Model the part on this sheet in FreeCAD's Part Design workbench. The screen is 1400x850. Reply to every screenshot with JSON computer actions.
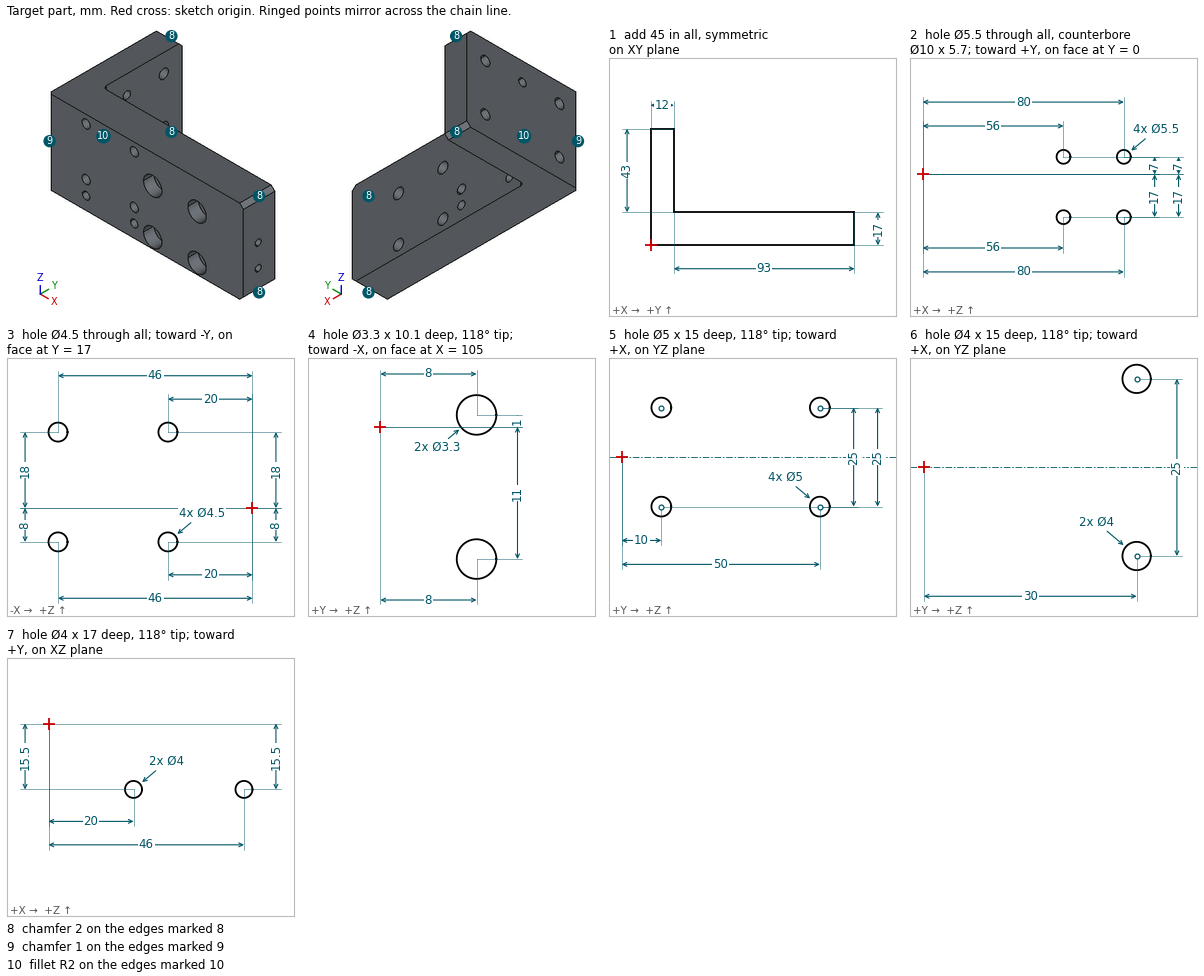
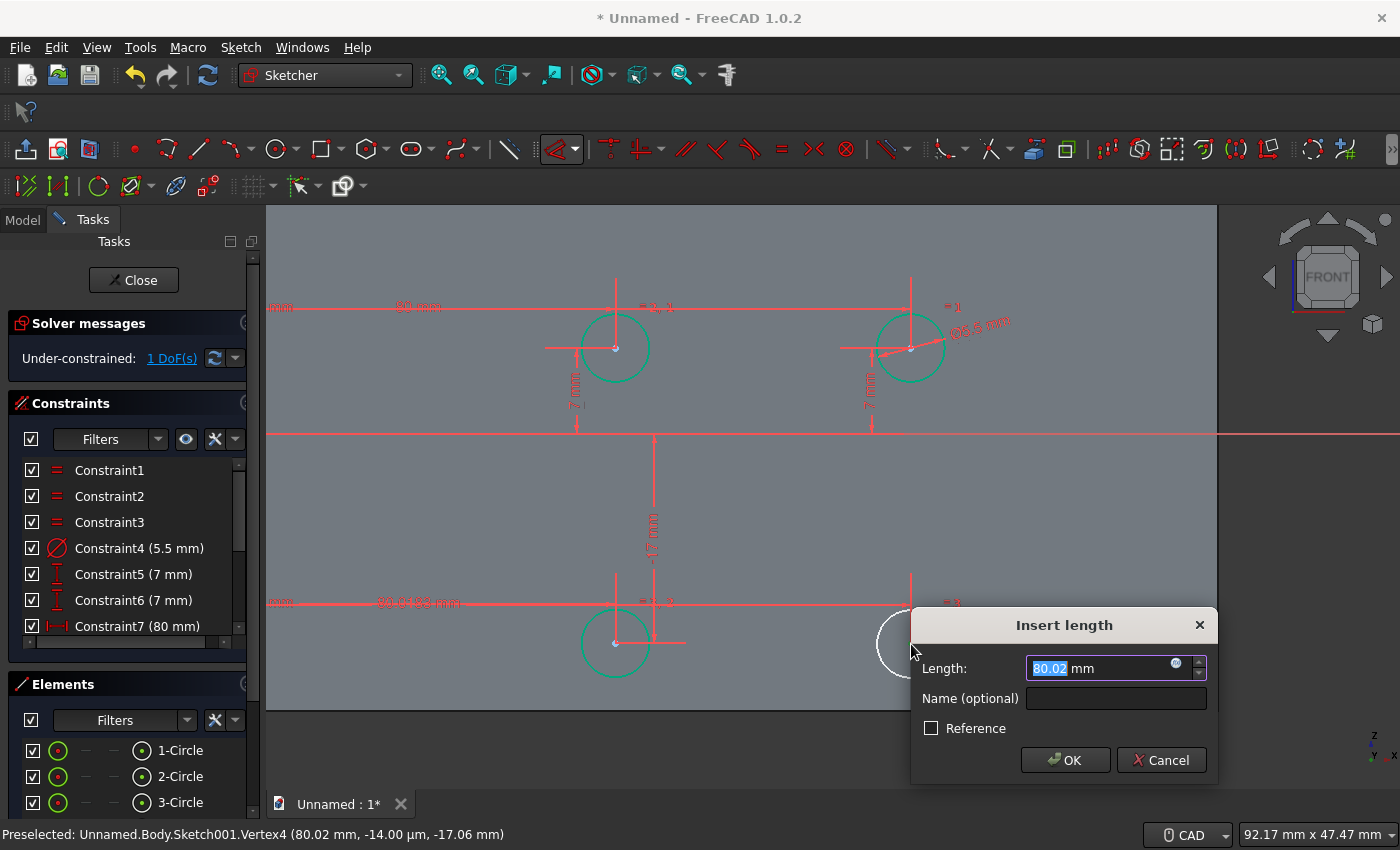
{"action": "type", "text": "80"}
{"action": "key", "text": "Return"}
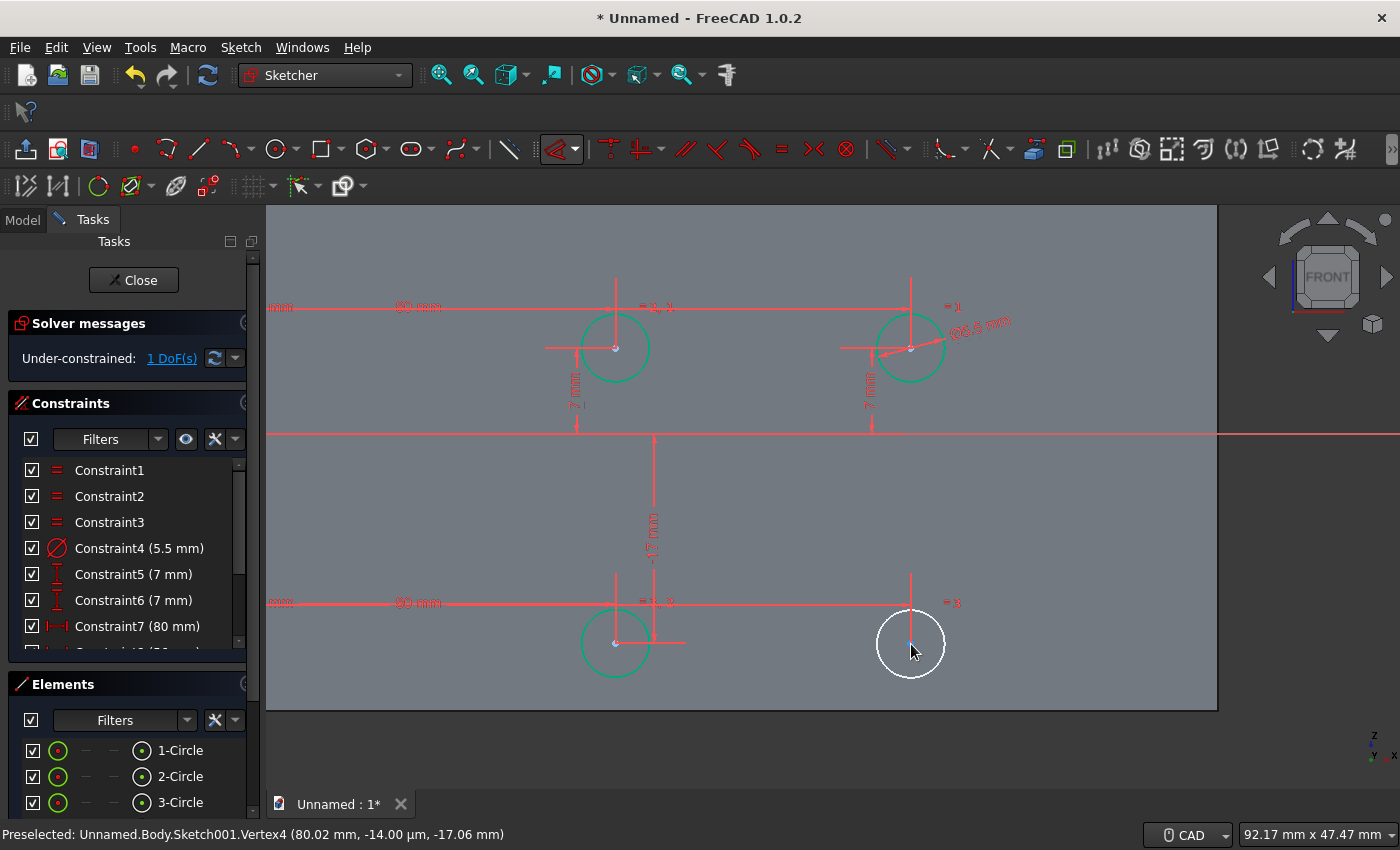
{"action": "left_click", "coordinate": [911, 644]}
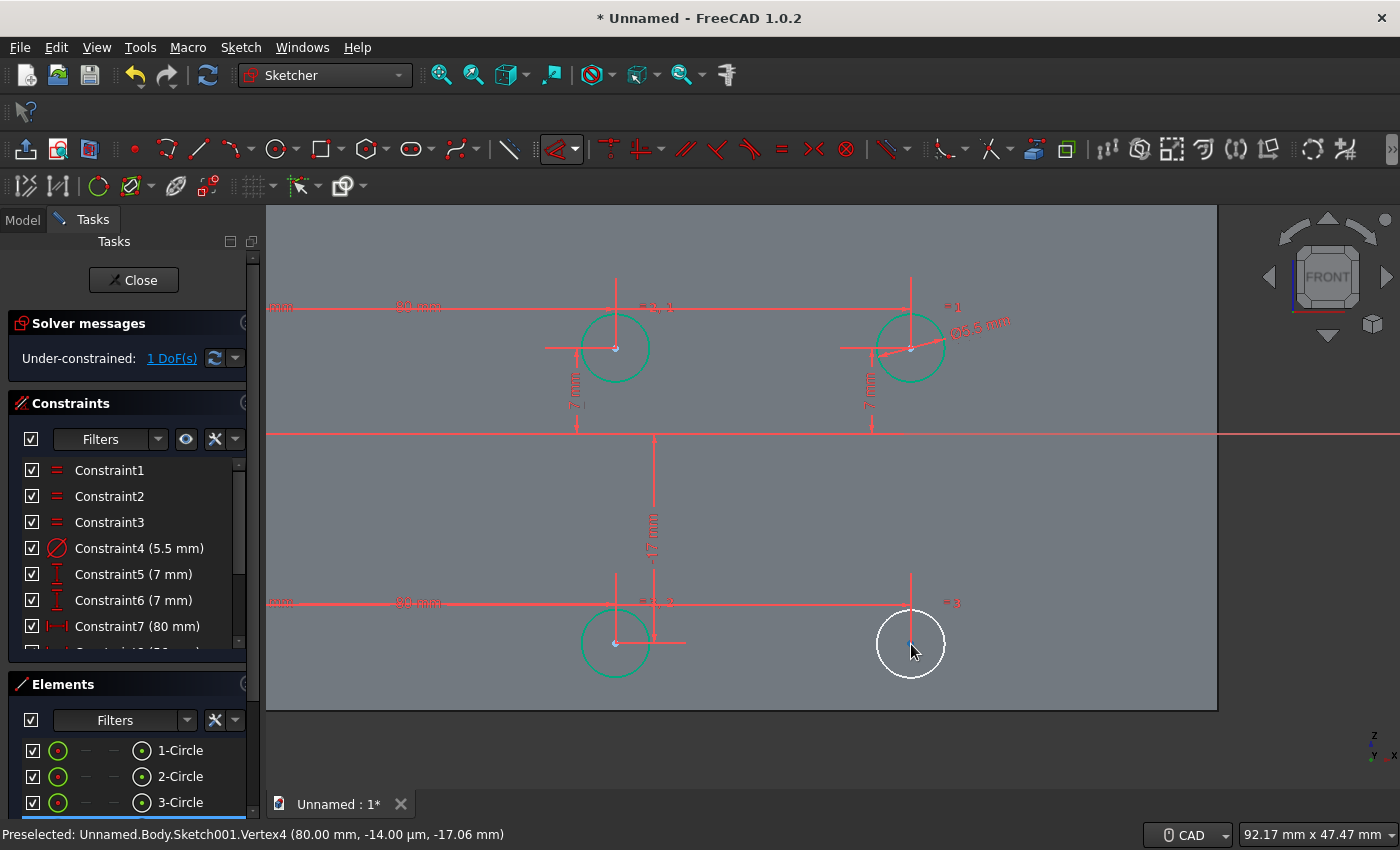
{"action": "key", "text": "i"}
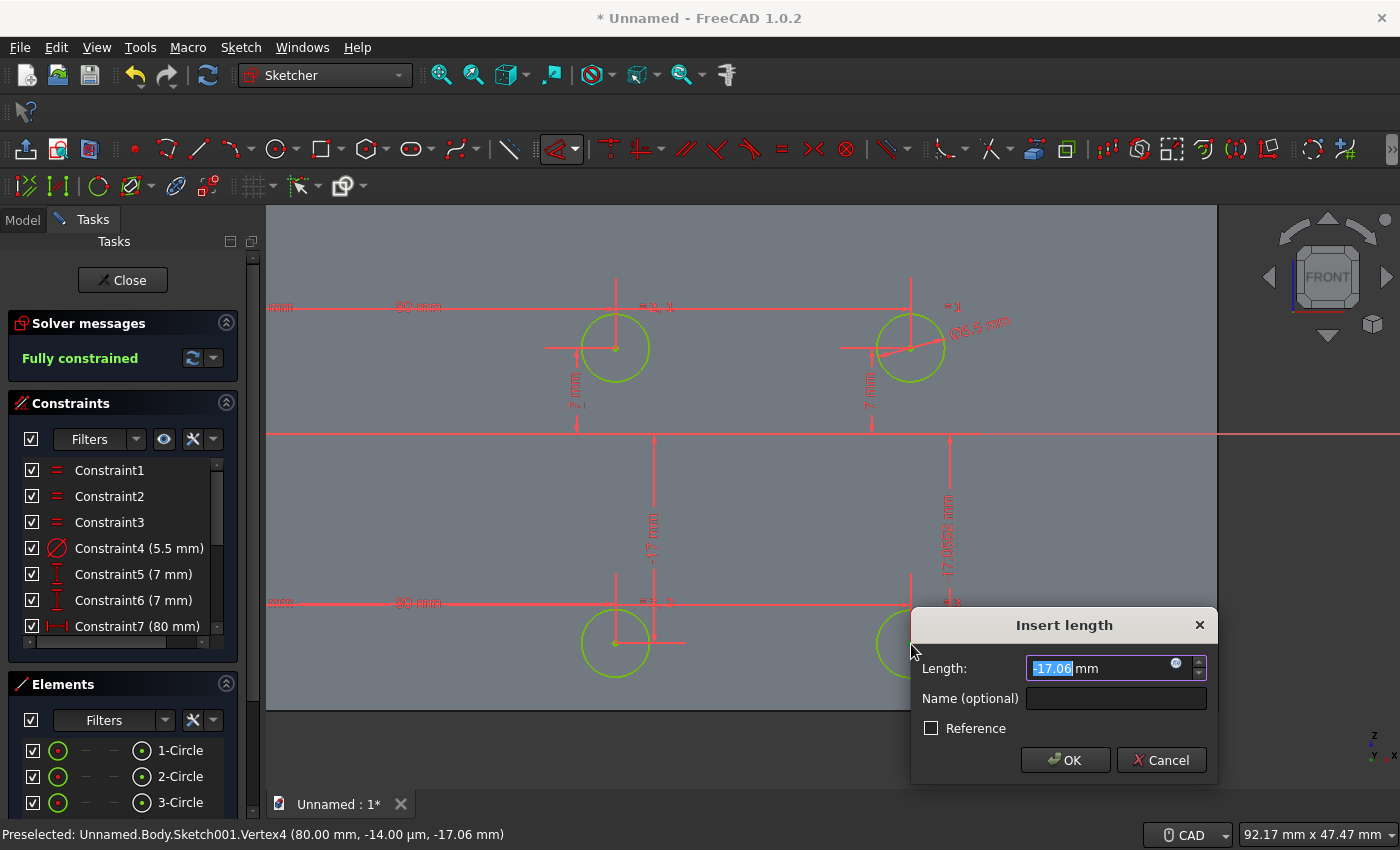
{"action": "type", "text": "-17"}
{"action": "key", "text": "Return"}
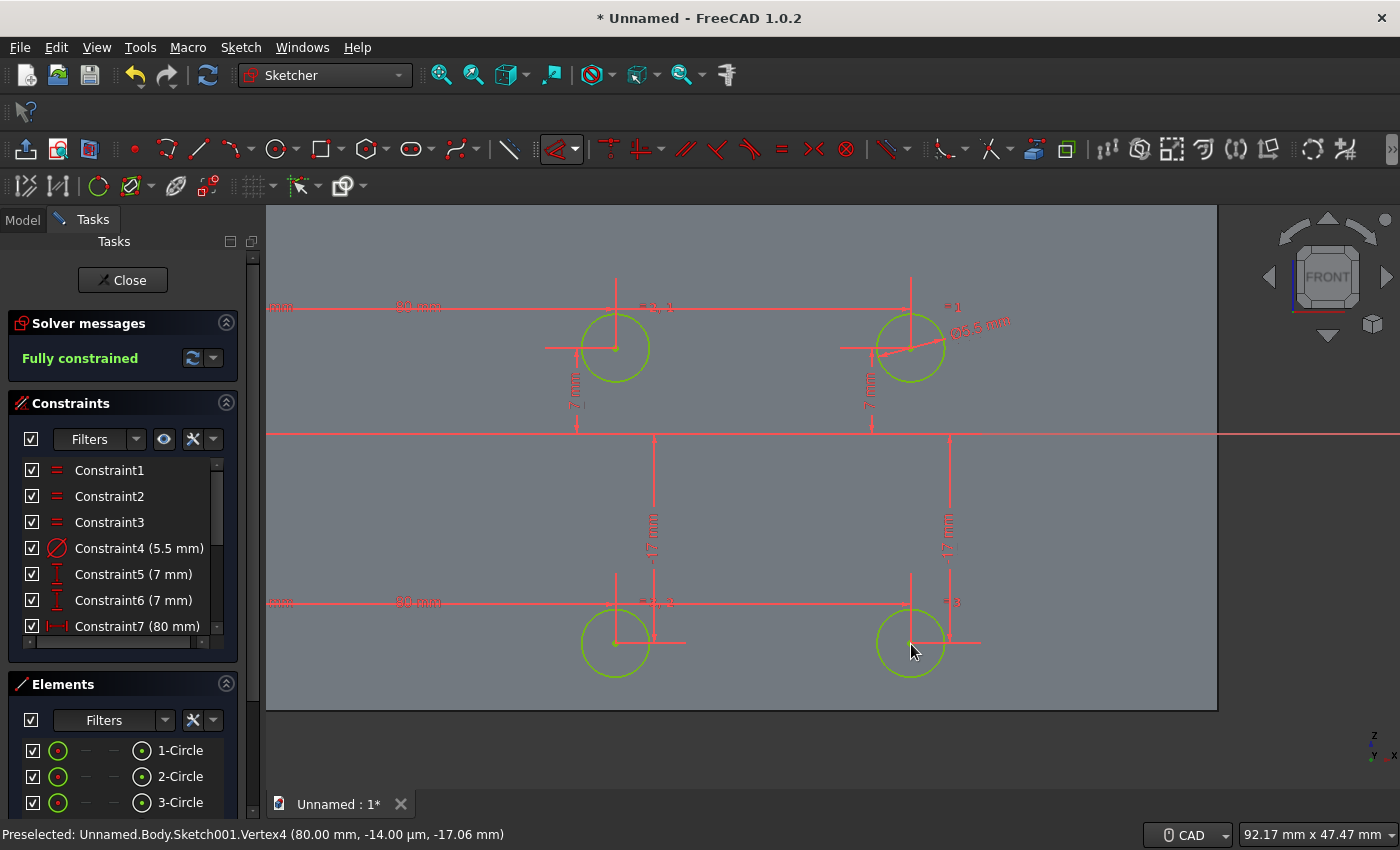
{"action": "left_click", "coordinate": [123, 280]}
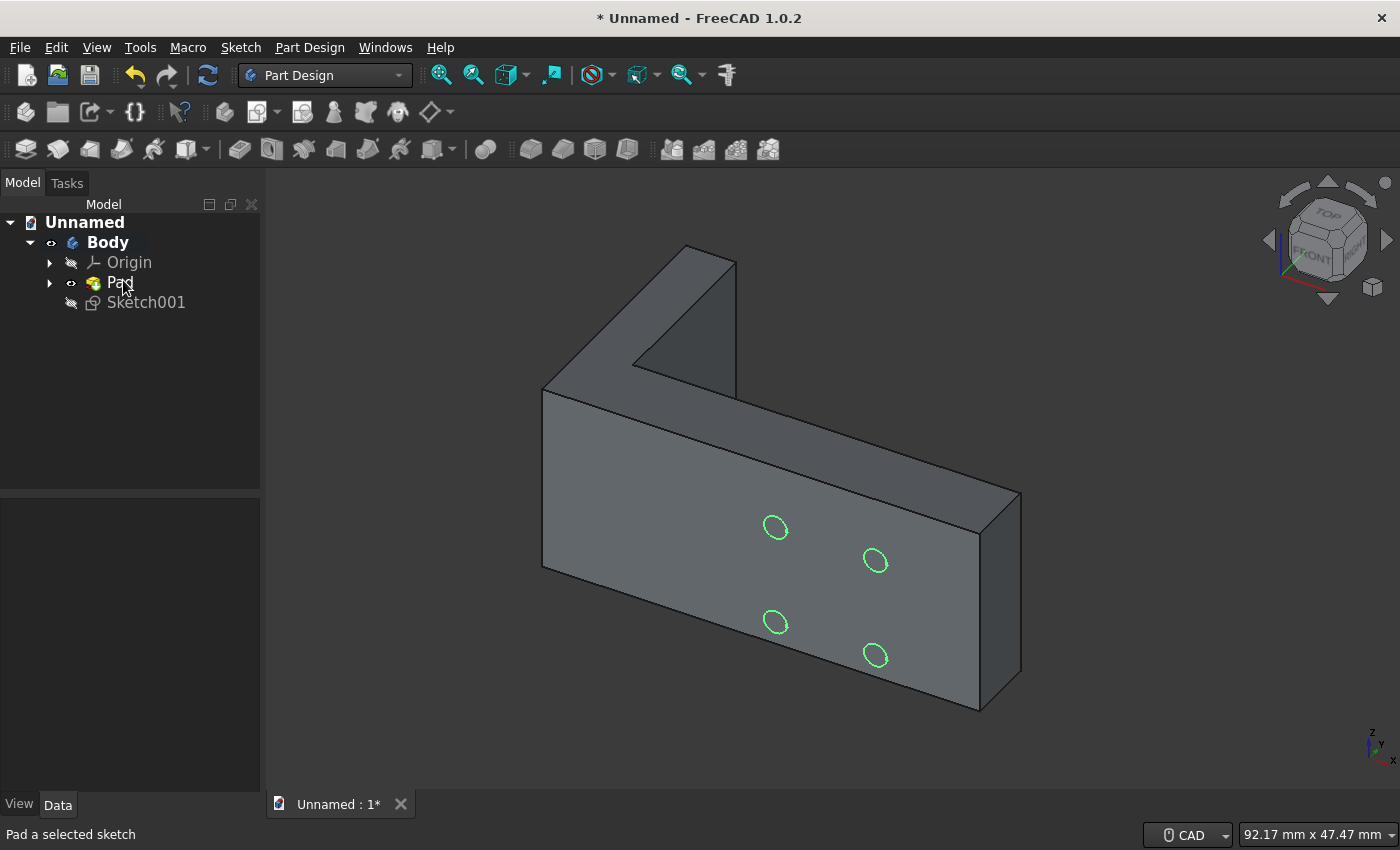
{"action": "left_click", "coordinate": [272, 150]}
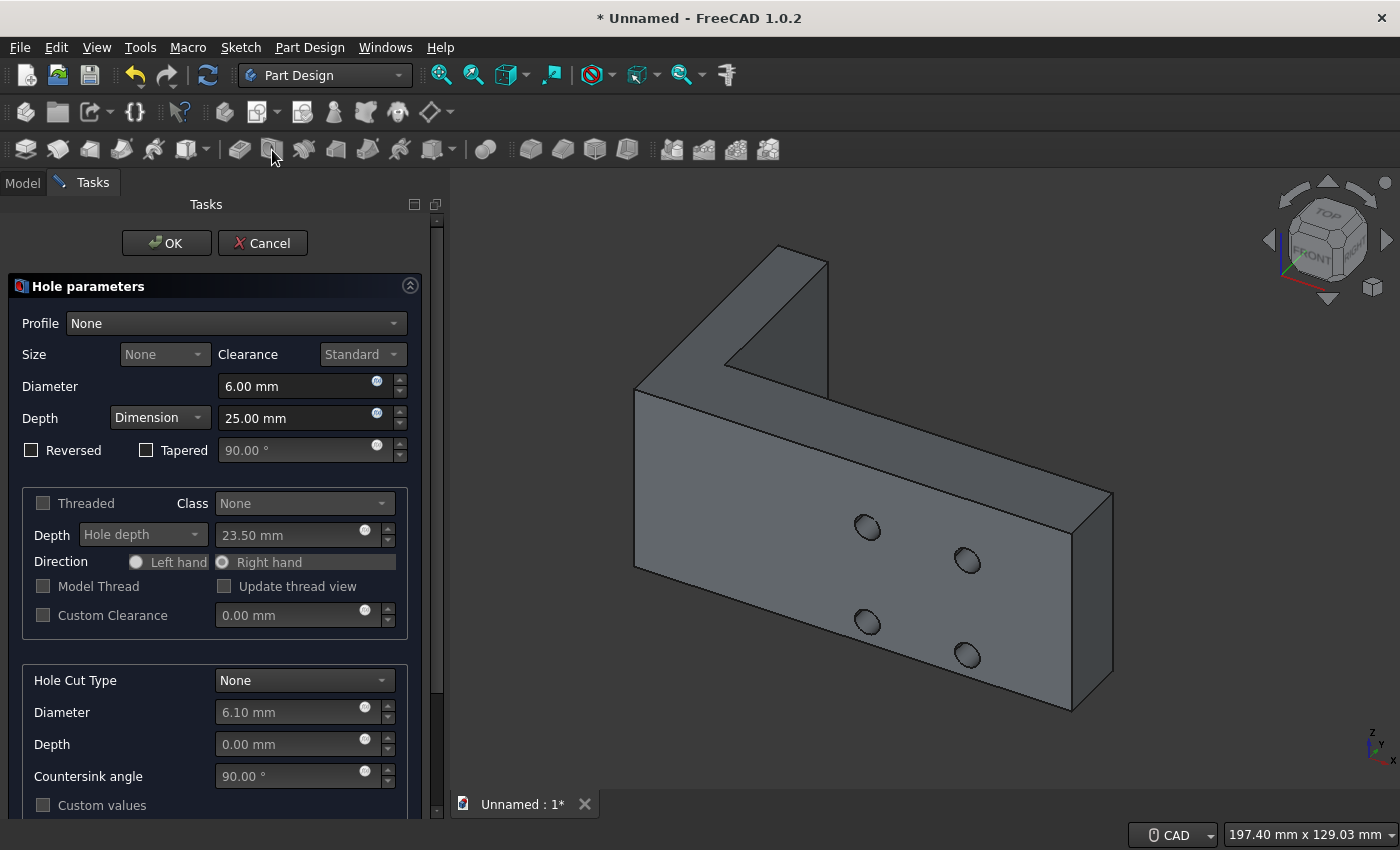
{"action": "triple_click", "coordinate": [305, 386]}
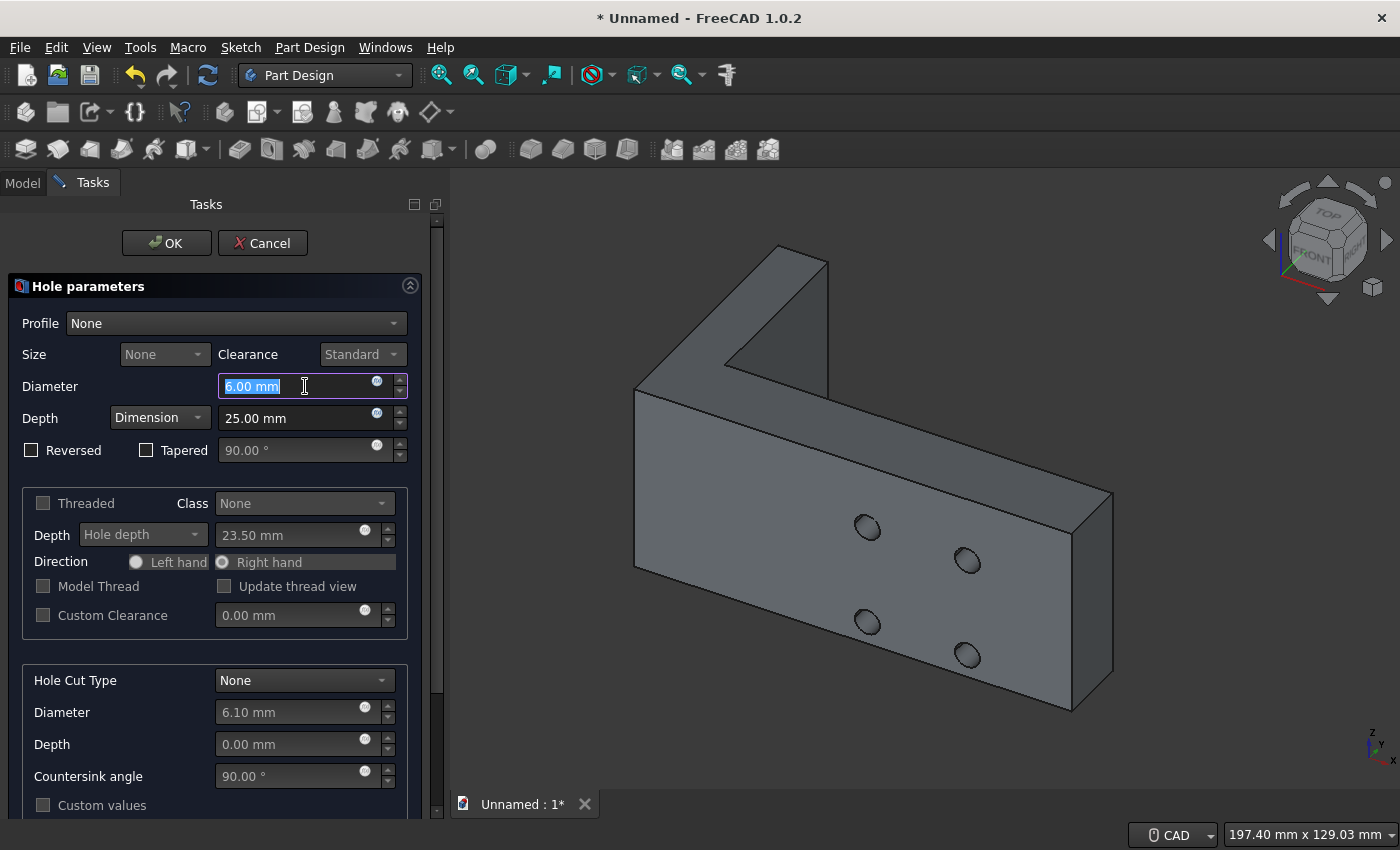
{"action": "type", "text": "5.5"}
{"action": "key", "text": "Tab"}